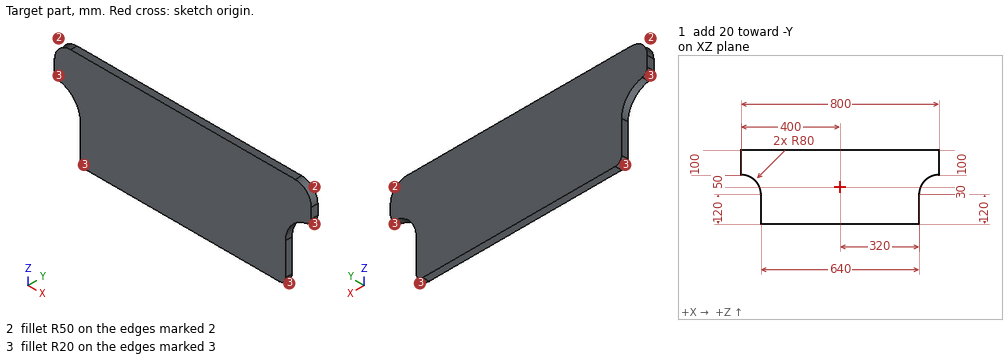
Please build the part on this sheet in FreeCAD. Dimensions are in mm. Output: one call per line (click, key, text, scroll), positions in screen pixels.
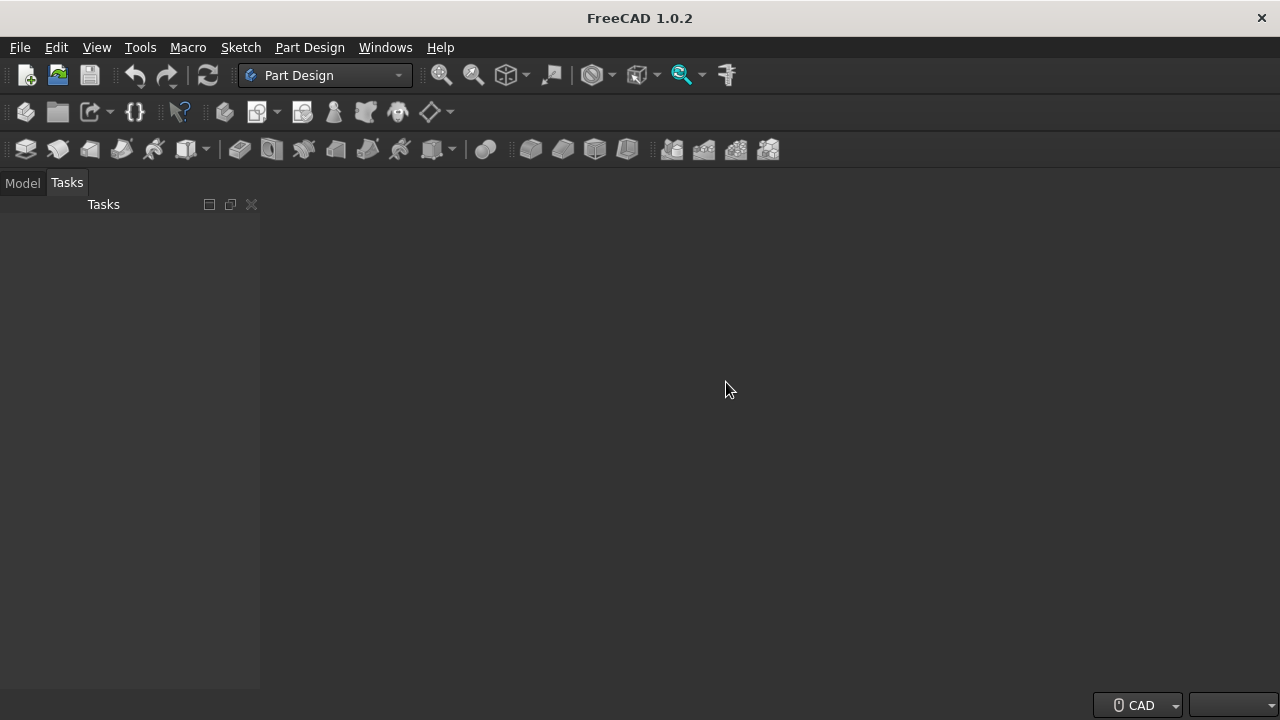
key(ctrl+n)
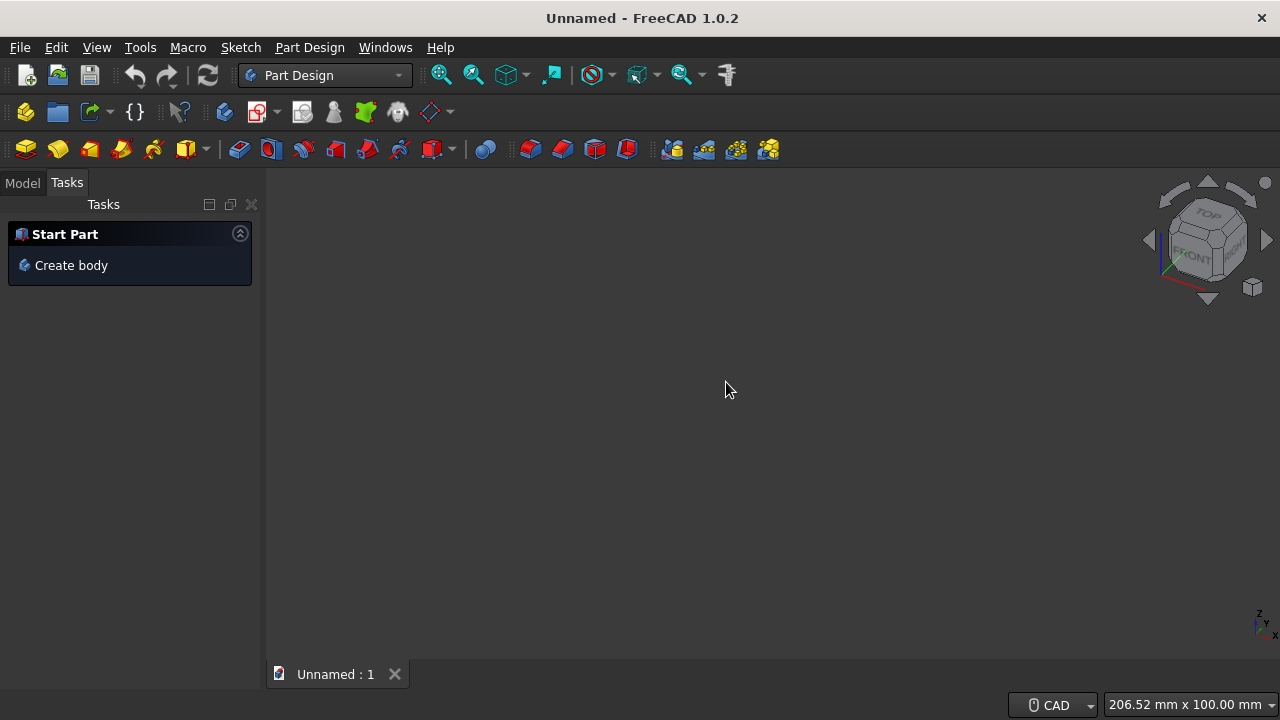
click(258, 112)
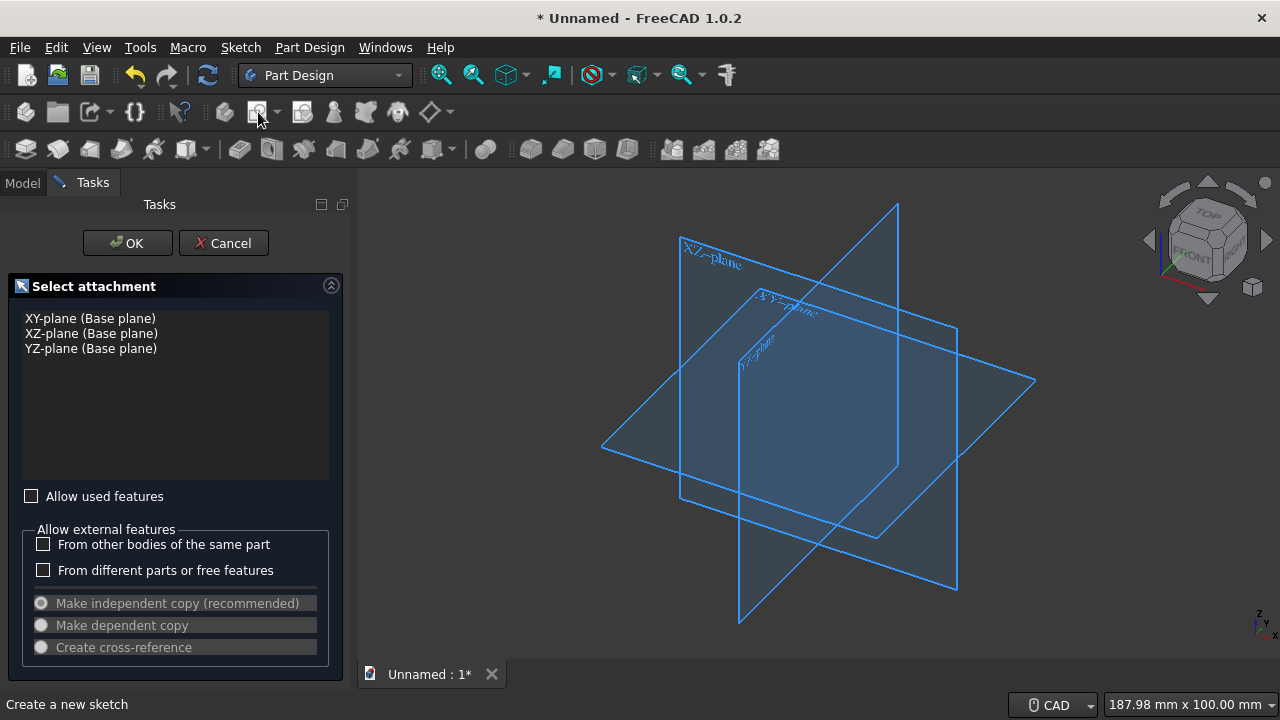
click(82, 334)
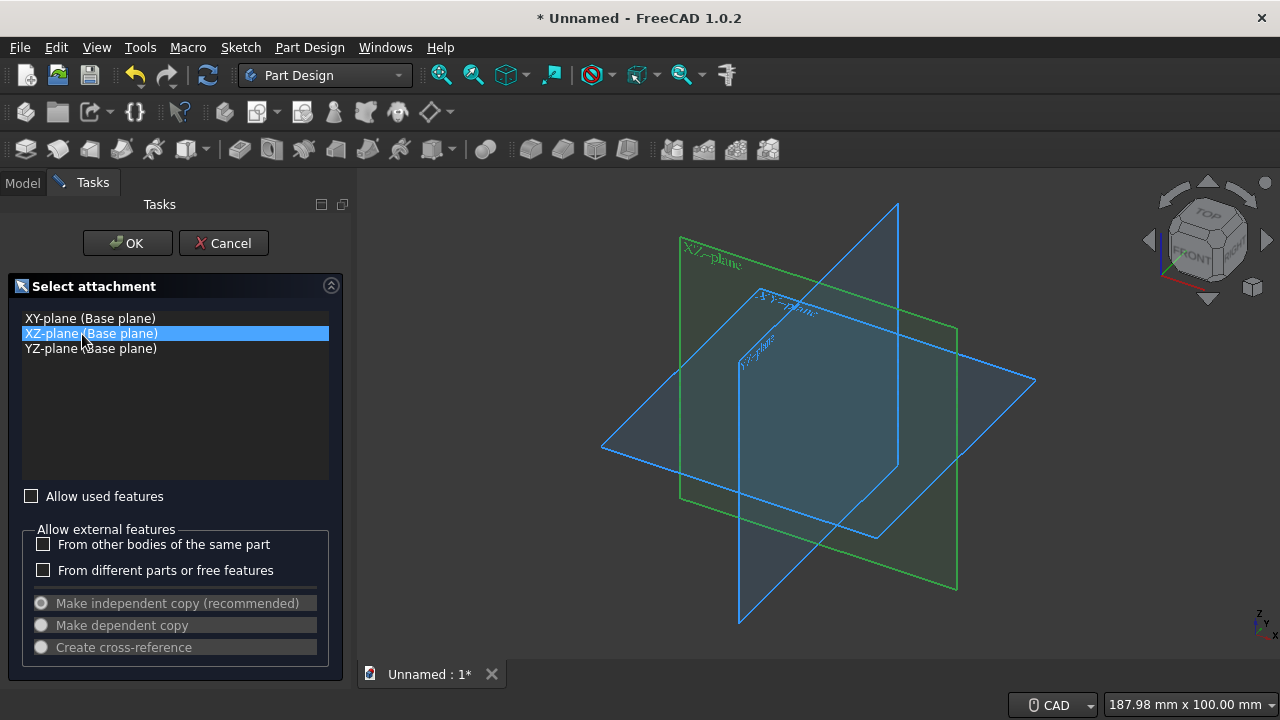
click(128, 243)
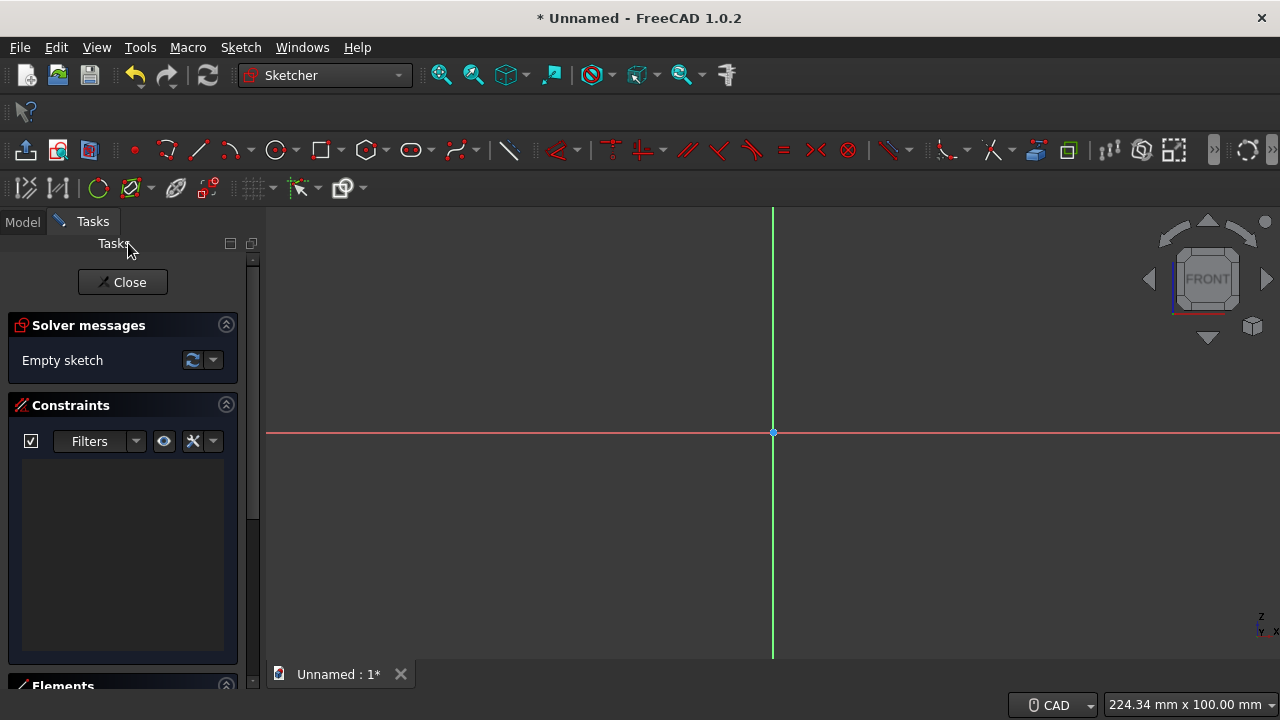
scroll(691, 433, down, 9)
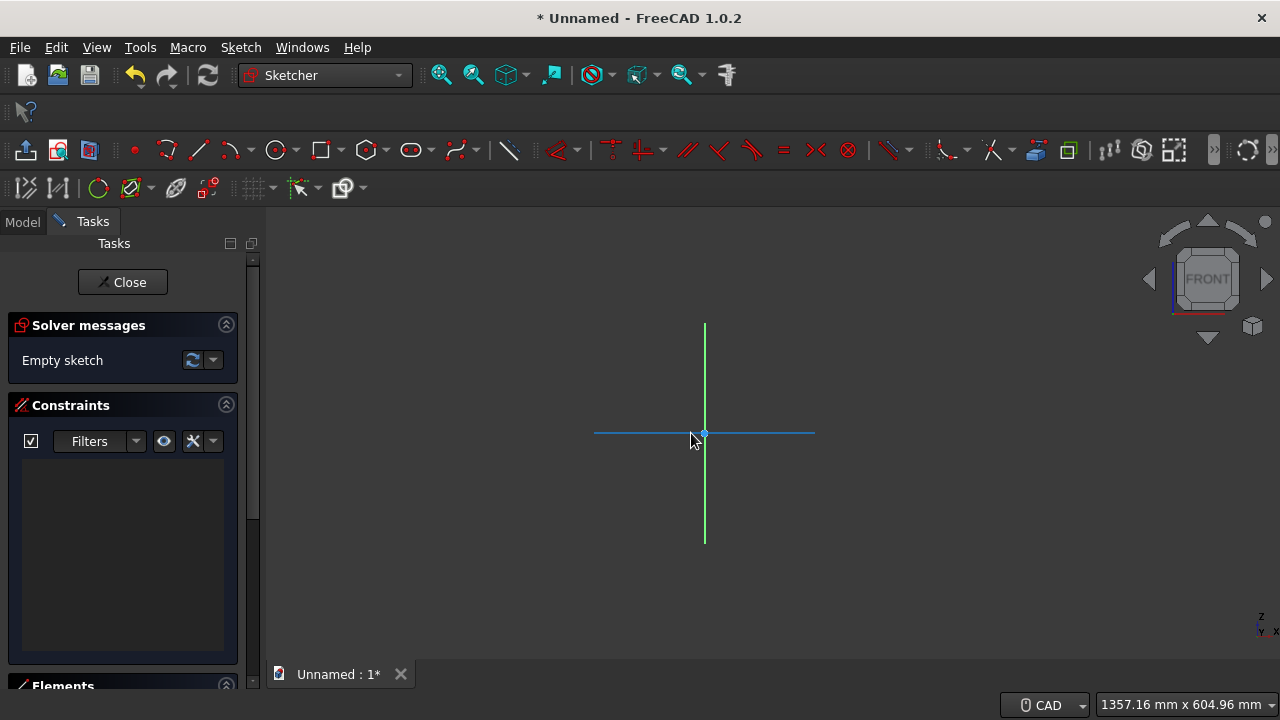
key(g)
key(m)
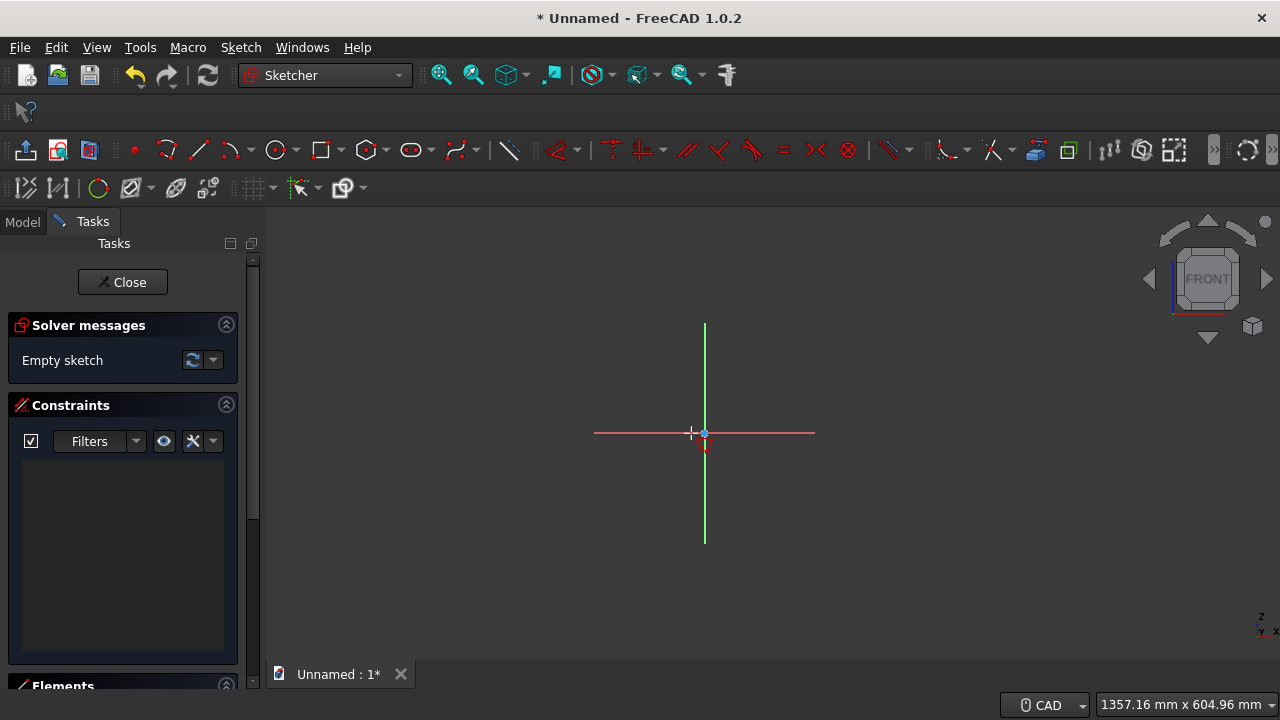
click(406, 396)
click(406, 321)
click(1004, 321)
click(1004, 396)
right_click(1004, 396)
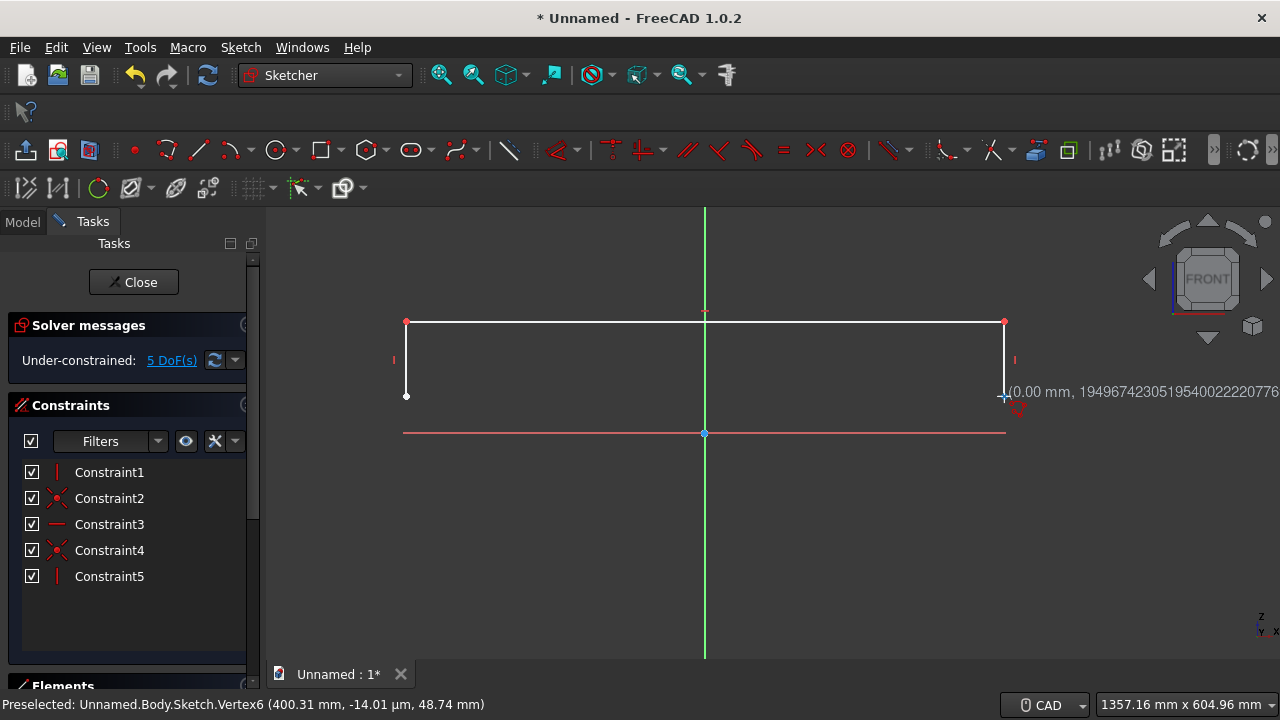
click(944, 456)
click(944, 545)
click(466, 545)
click(466, 456)
right_click(466, 456)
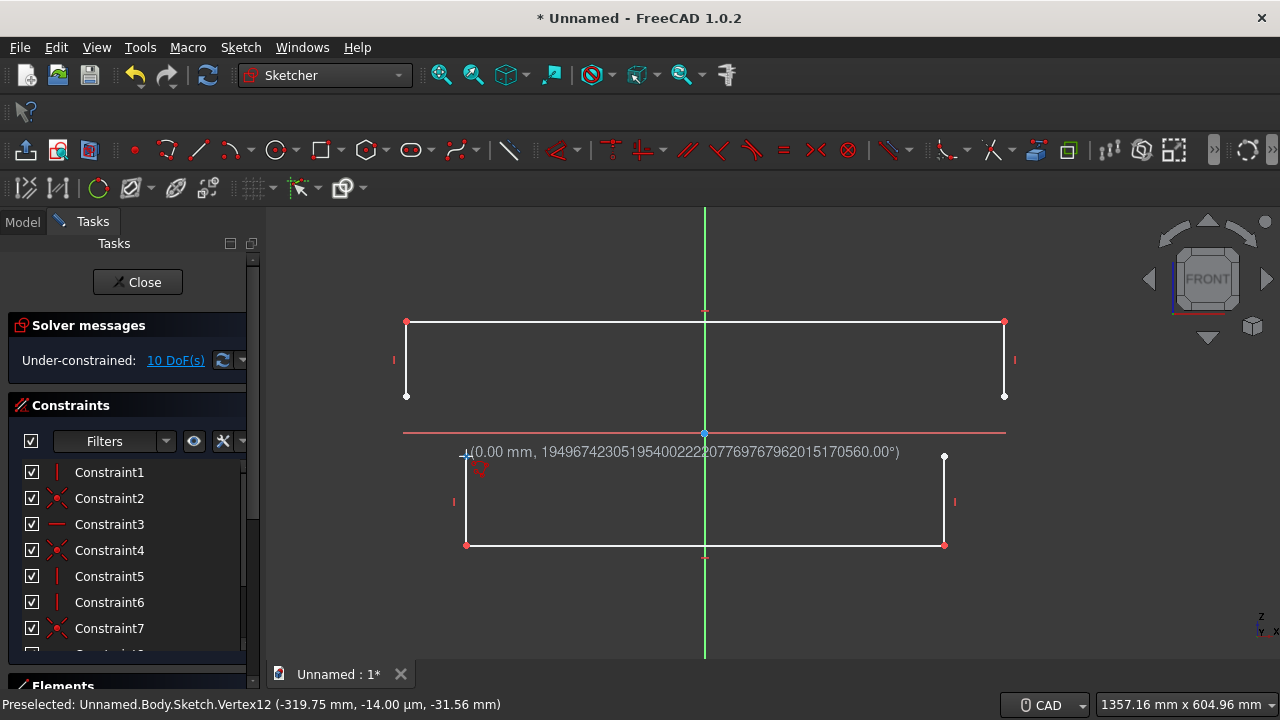
key(g)
key(3)
key(a)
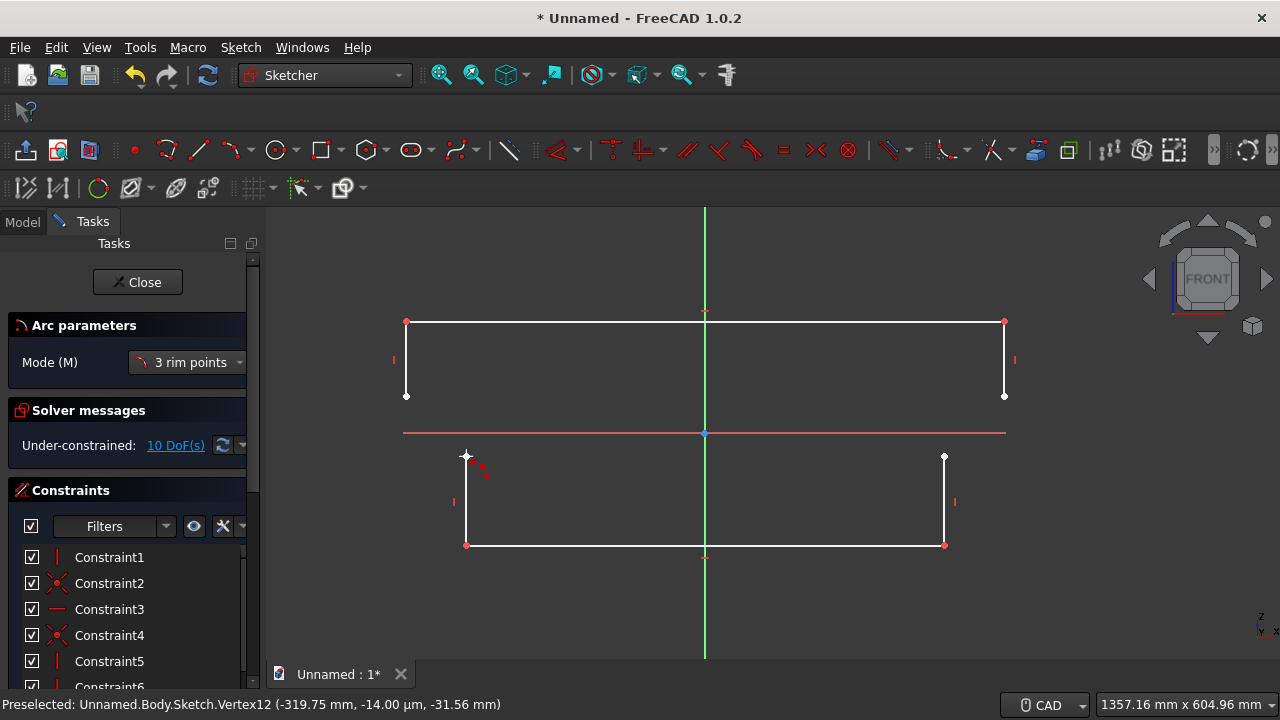
click(1004, 397)
click(944, 457)
click(961, 414)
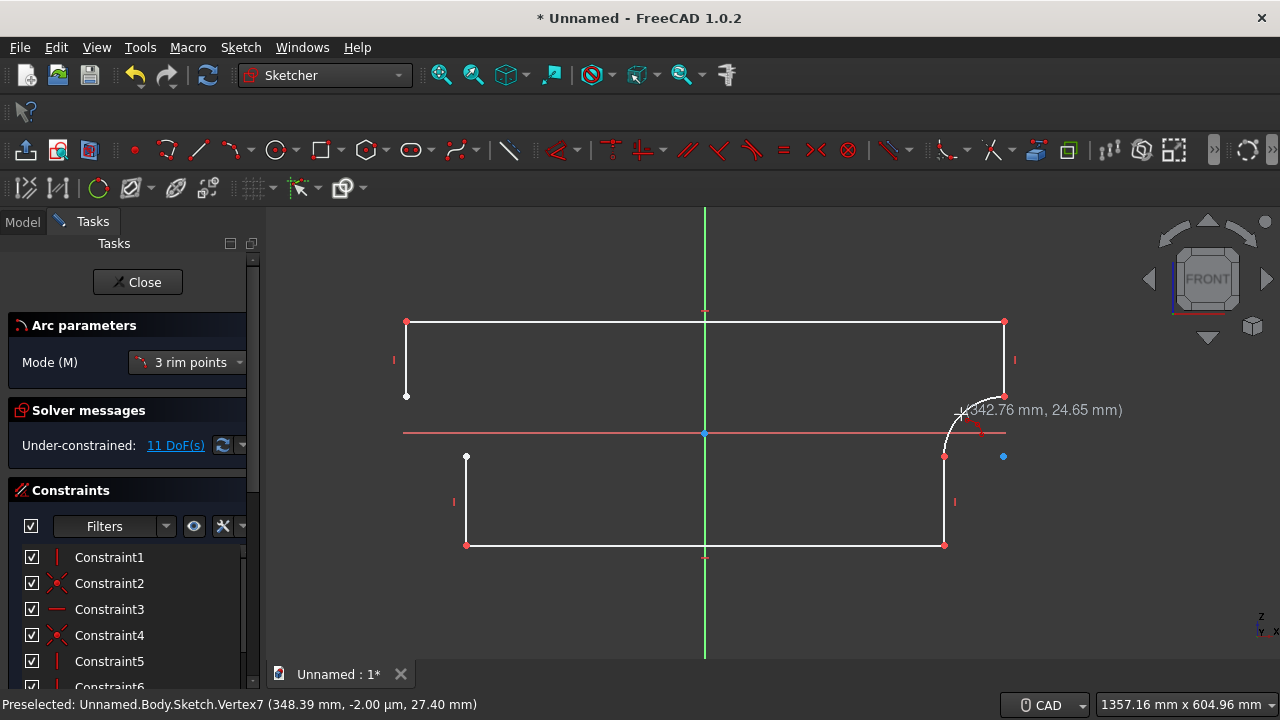
click(466, 457)
click(406, 397)
click(448, 414)
key(Escape)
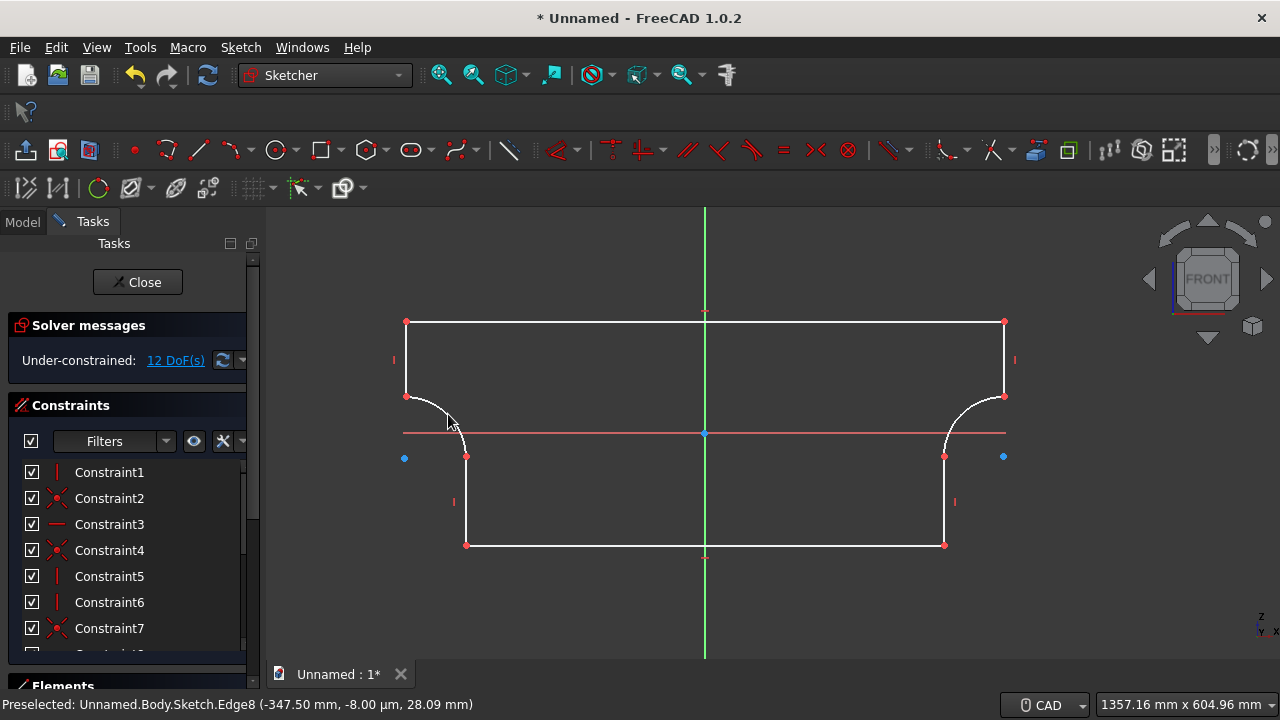
click(977, 403)